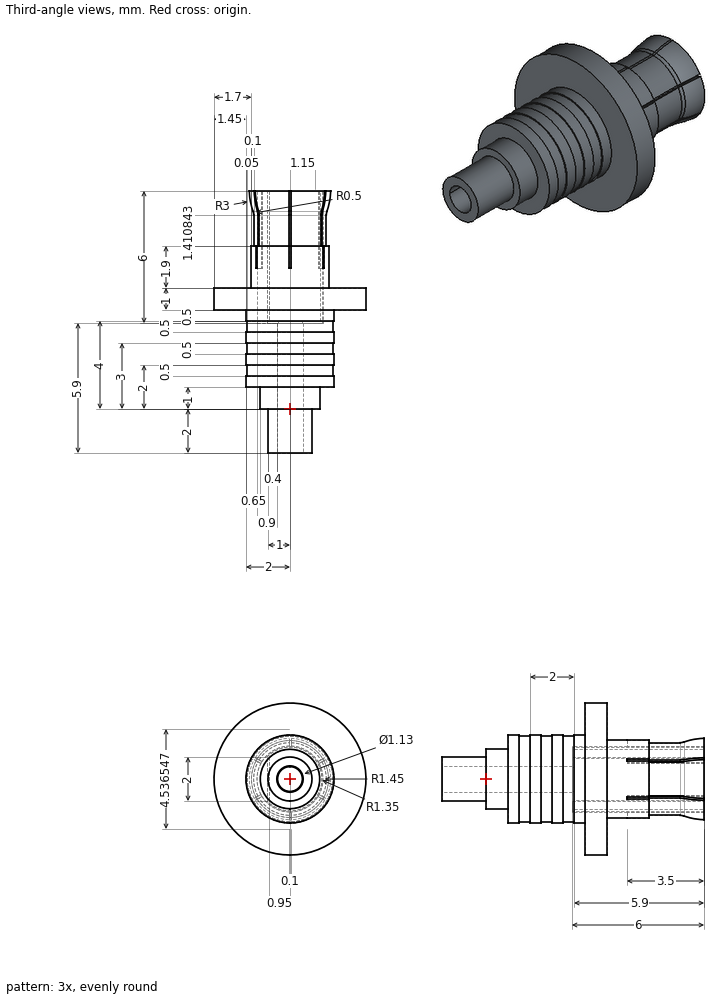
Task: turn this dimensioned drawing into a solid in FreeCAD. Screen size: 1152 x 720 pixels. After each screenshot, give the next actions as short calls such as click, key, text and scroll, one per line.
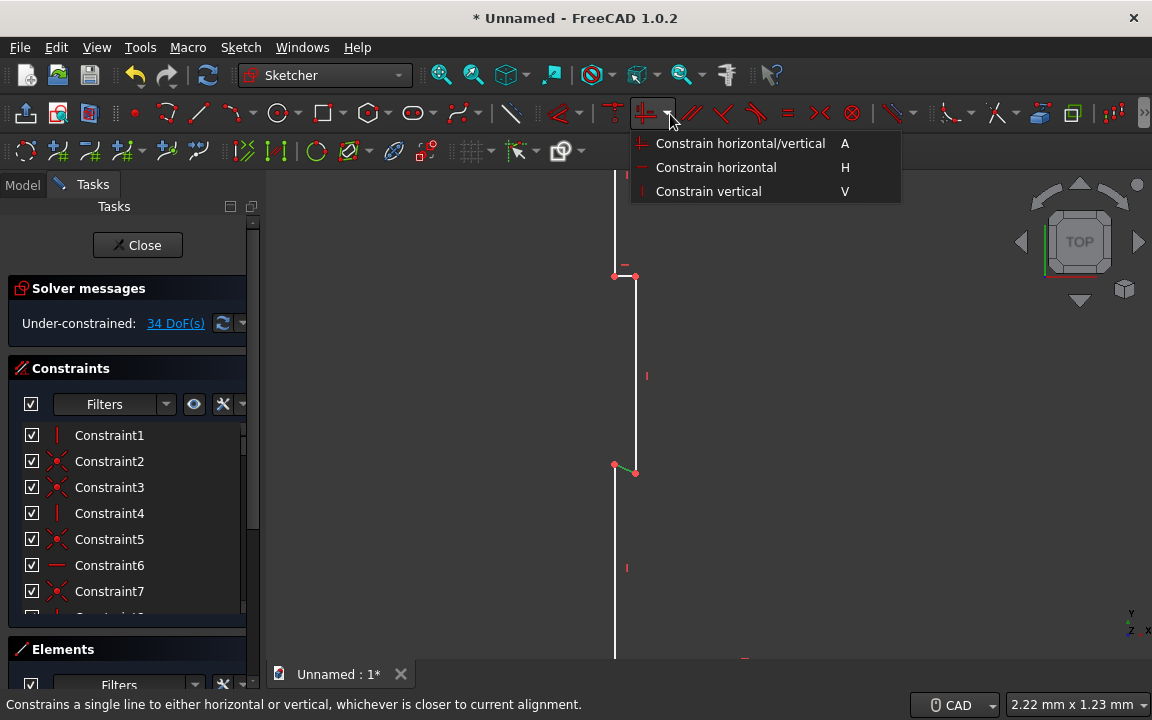
click(766, 167)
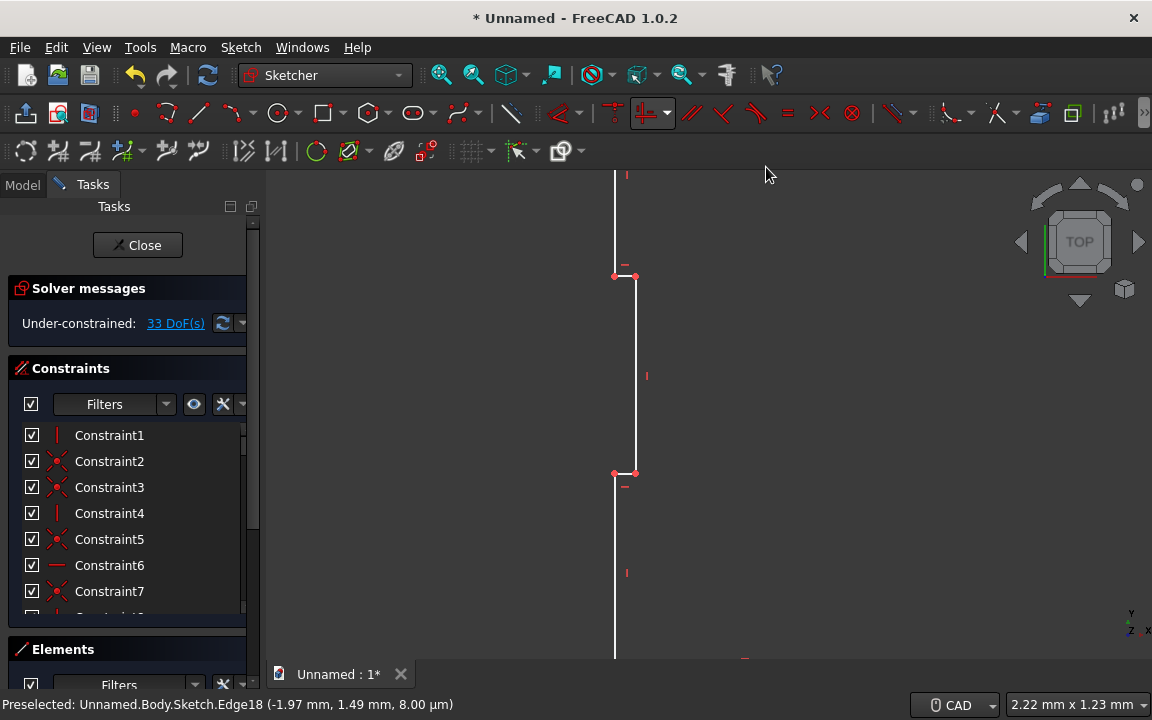
scroll(635, 474, down, 14)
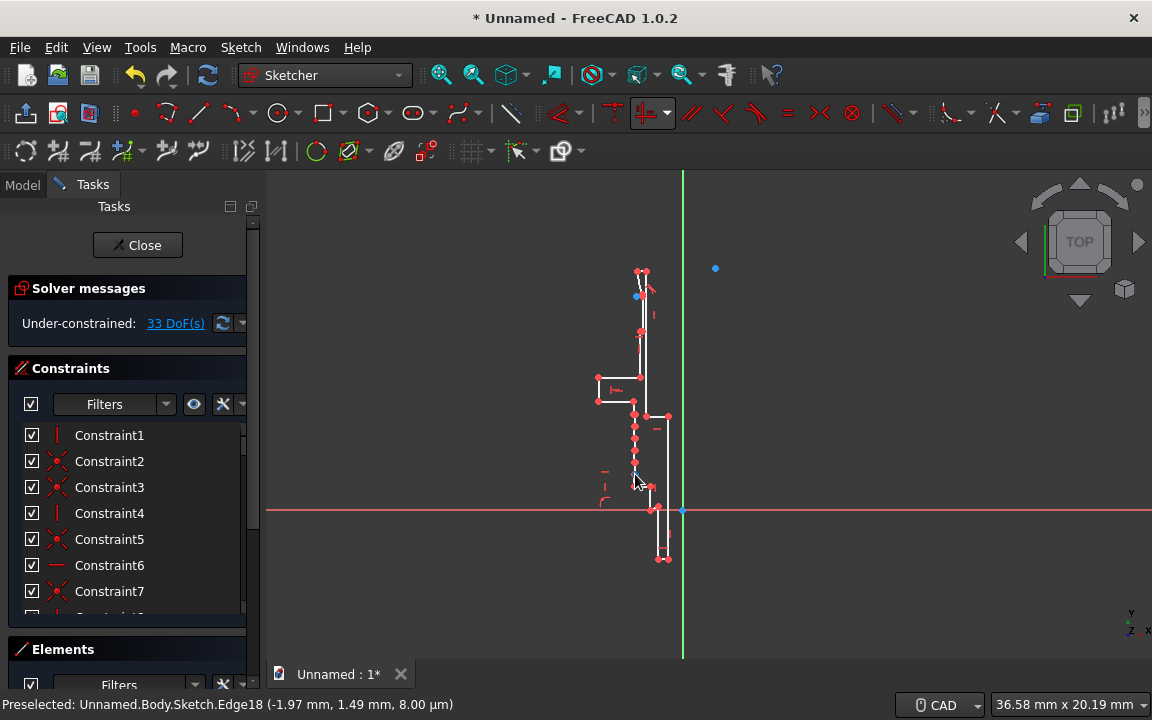
scroll(653, 509, up, 13)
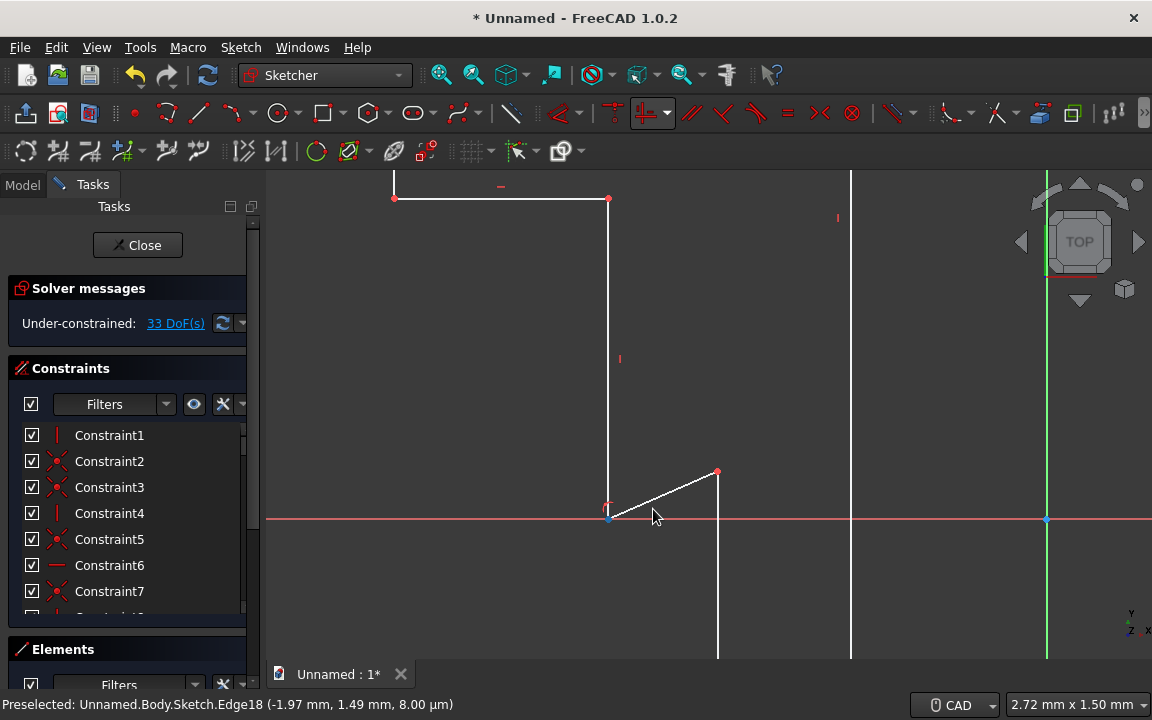
click(641, 505)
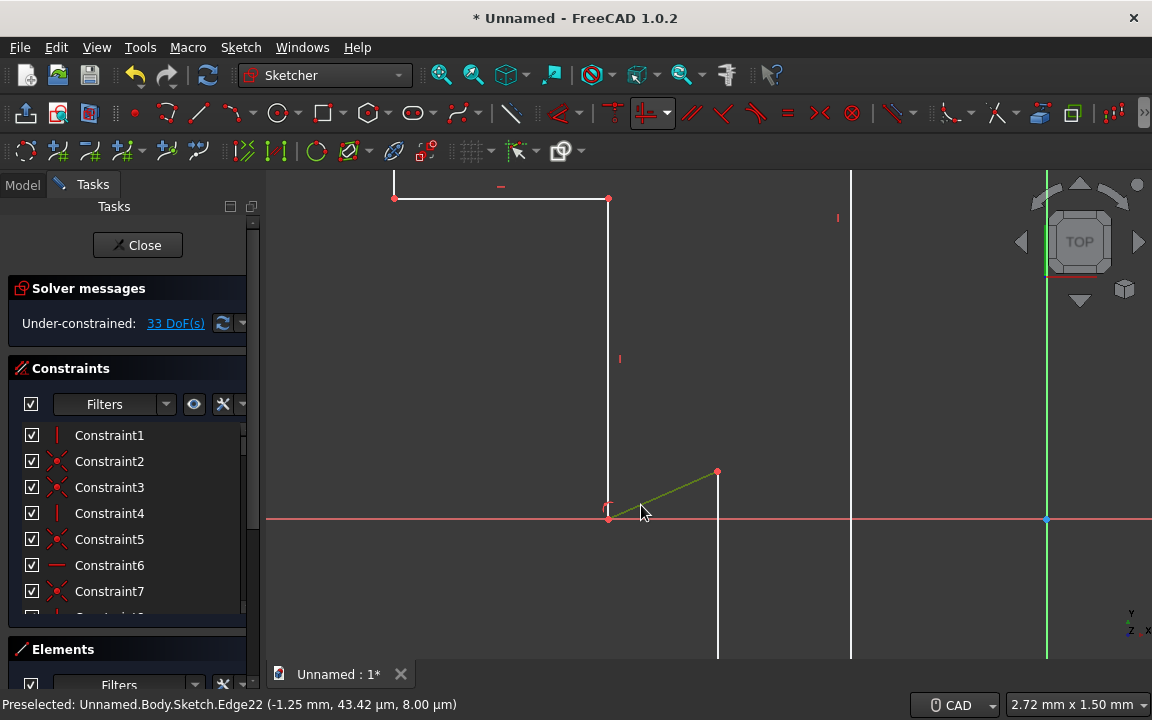
key(h)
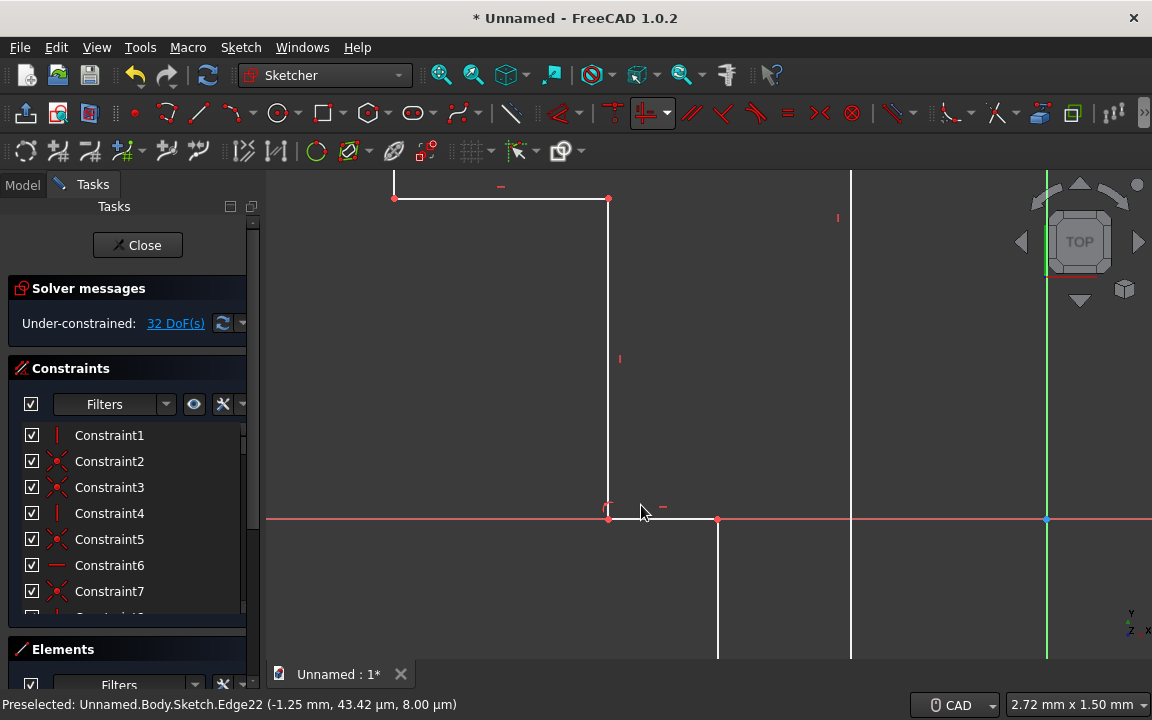
scroll(653, 509, down, 13)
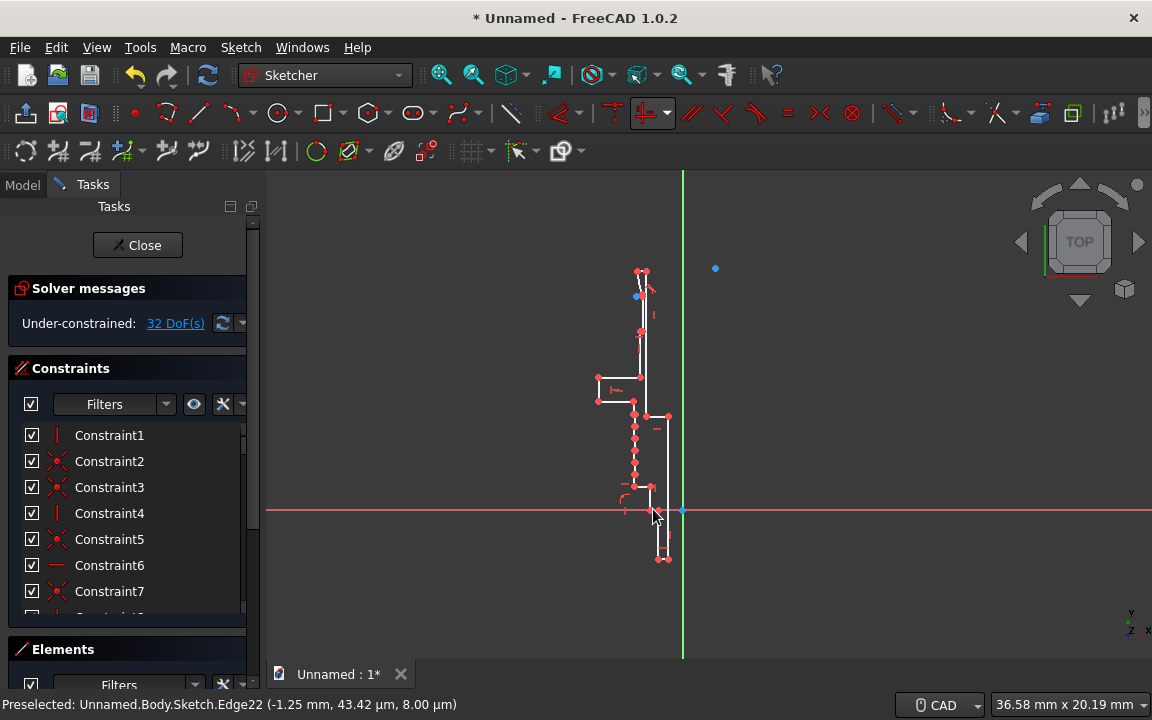
scroll(644, 271, up, 9)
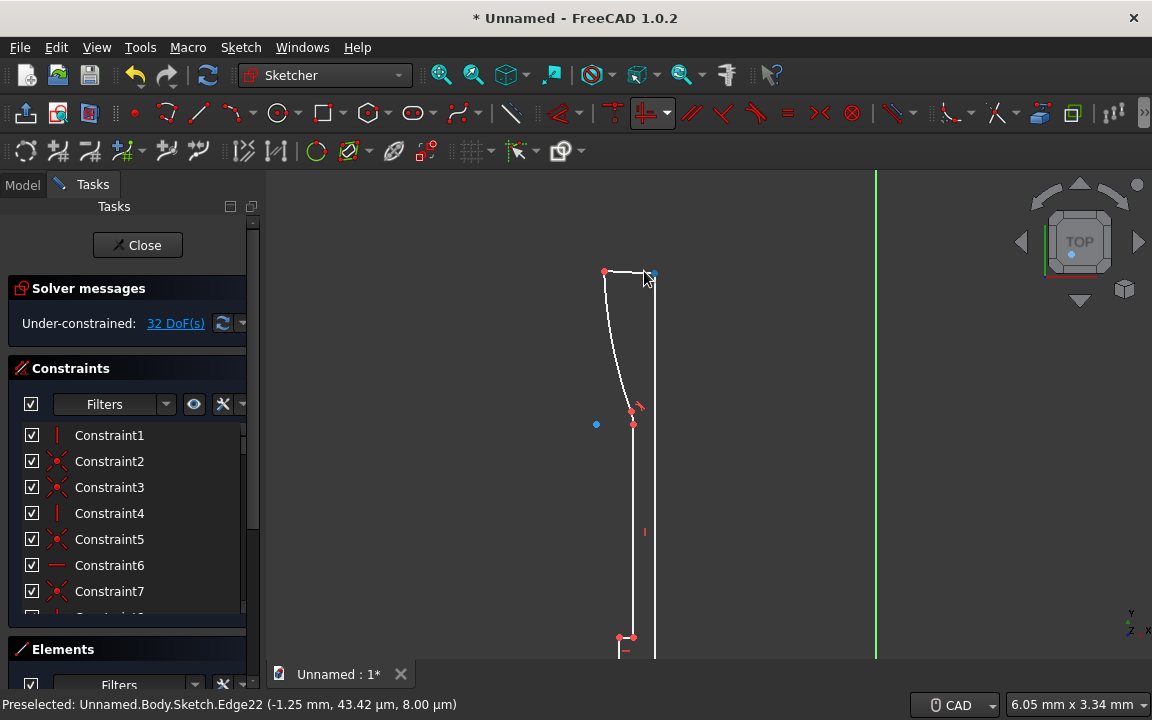
click(639, 273)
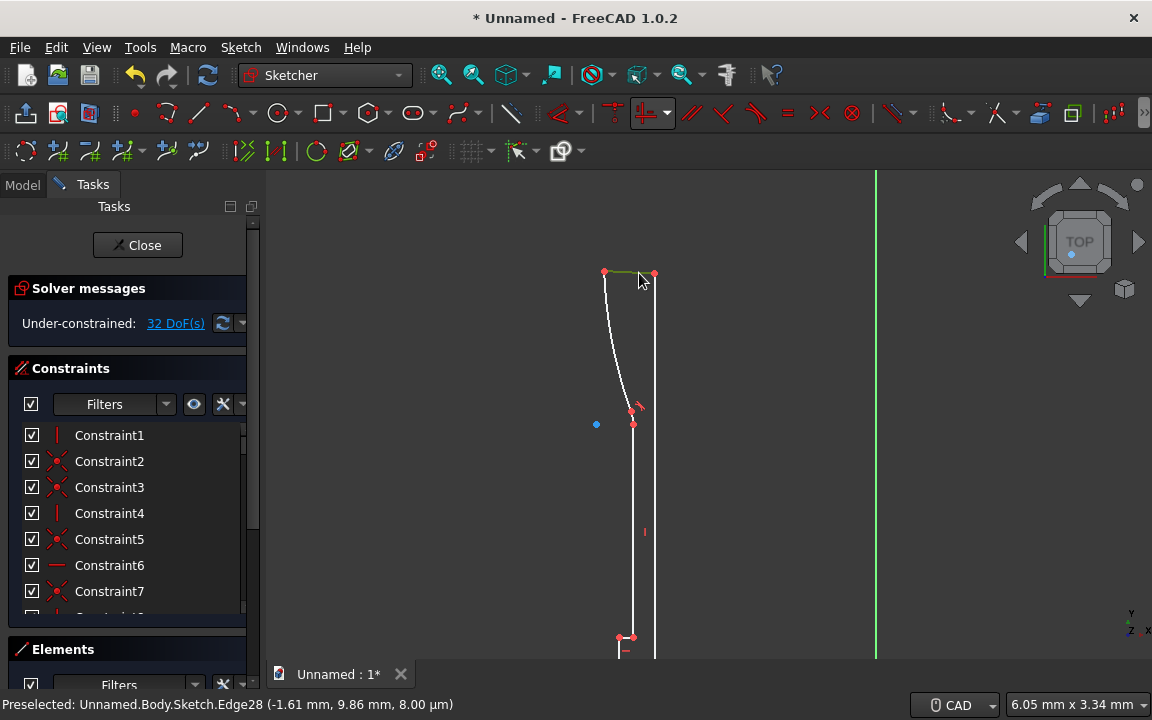
click(670, 114)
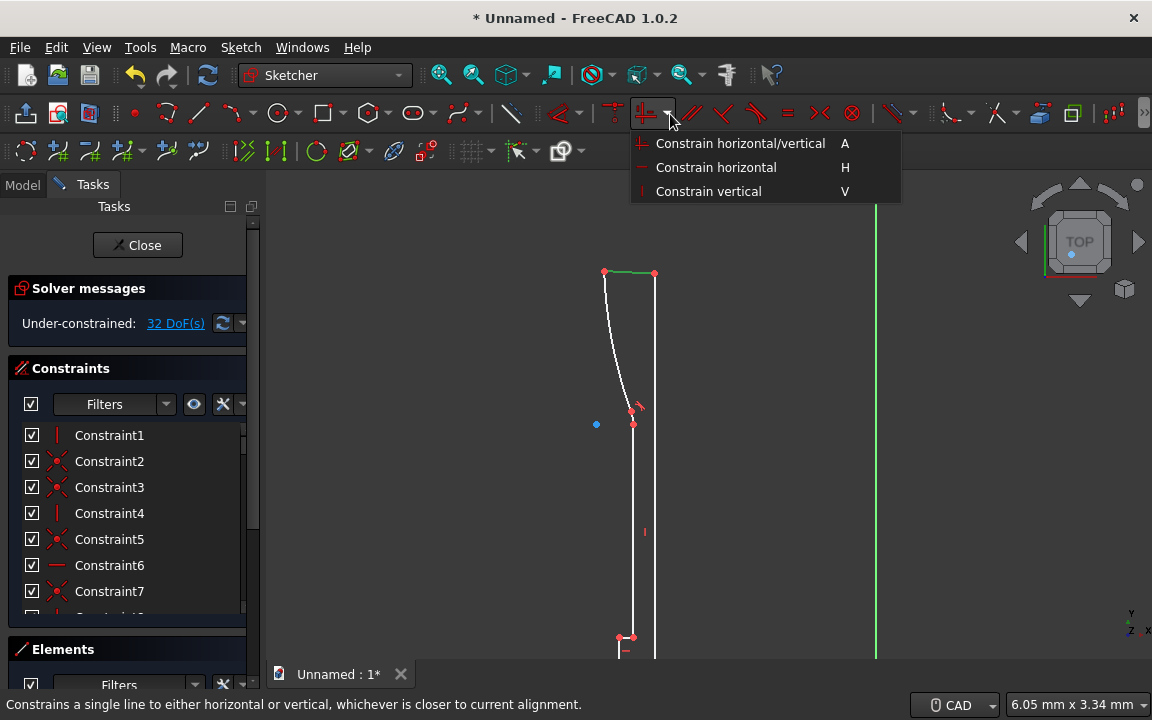
click(766, 167)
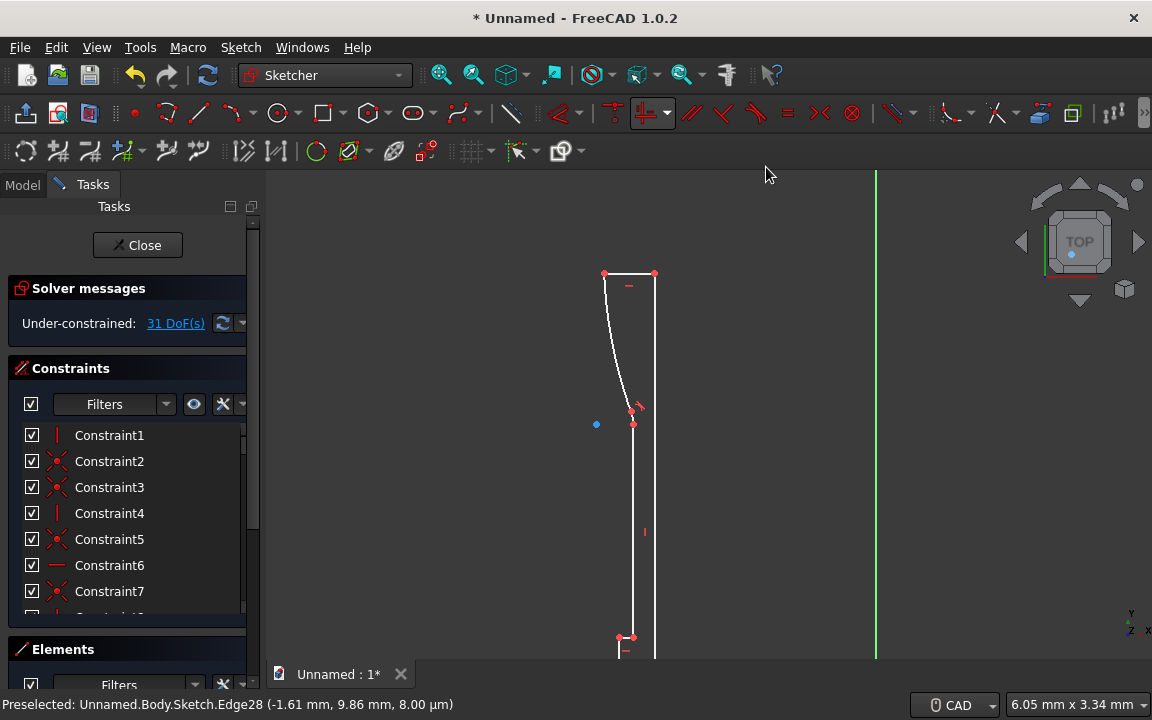
click(558, 114)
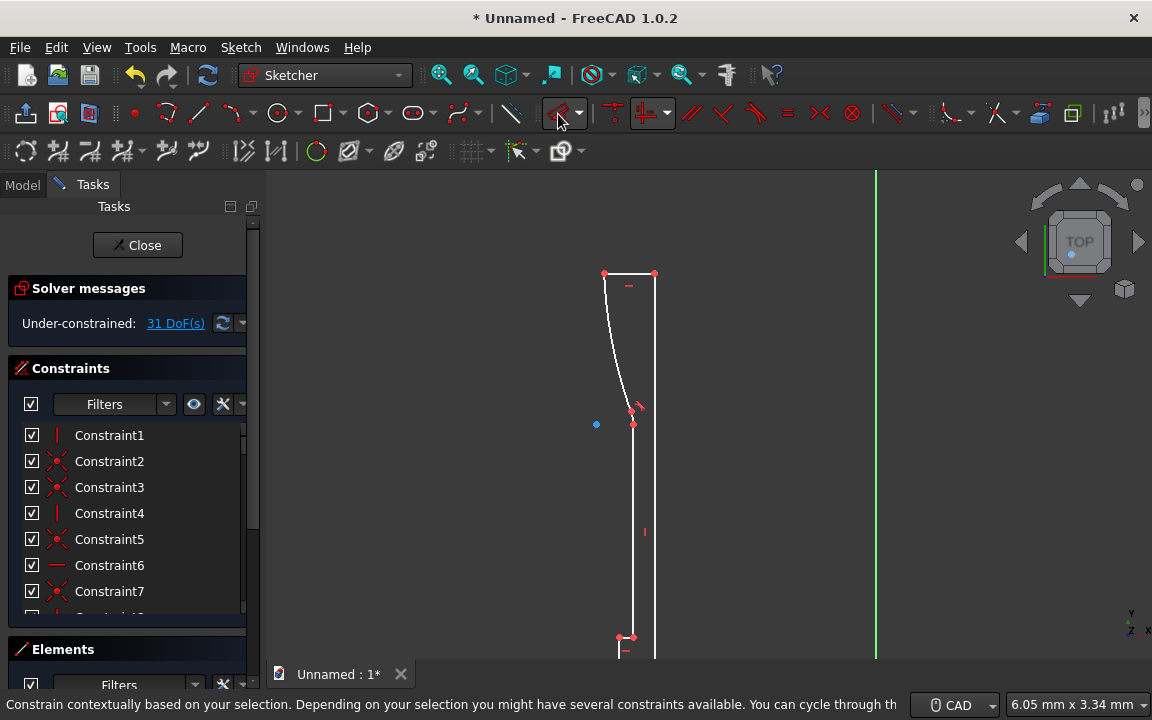
scroll(644, 271, down, 9)